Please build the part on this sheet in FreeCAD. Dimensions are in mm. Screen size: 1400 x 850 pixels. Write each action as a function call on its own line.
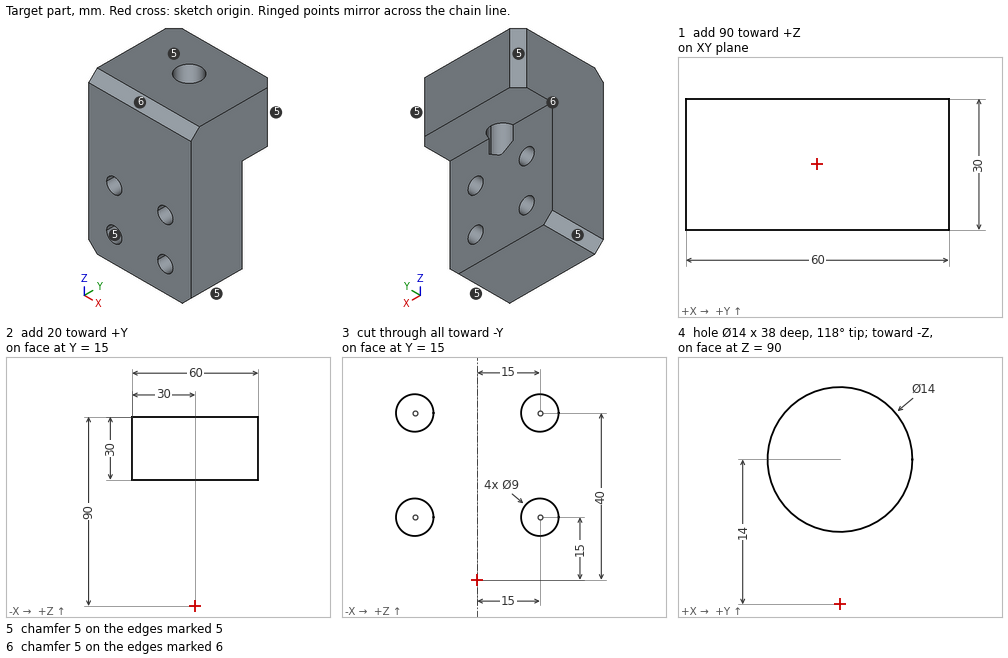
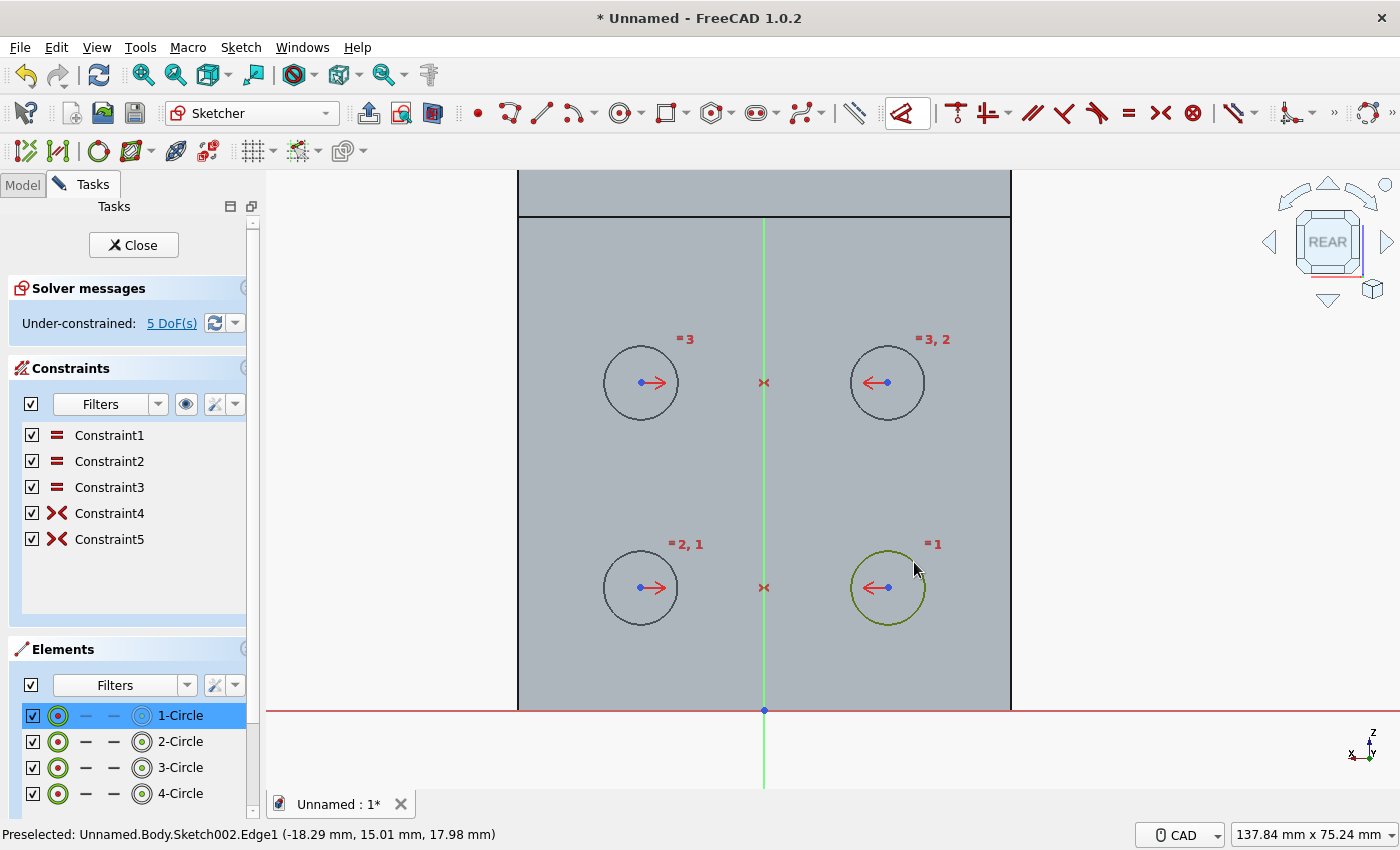
key(k)
key(o)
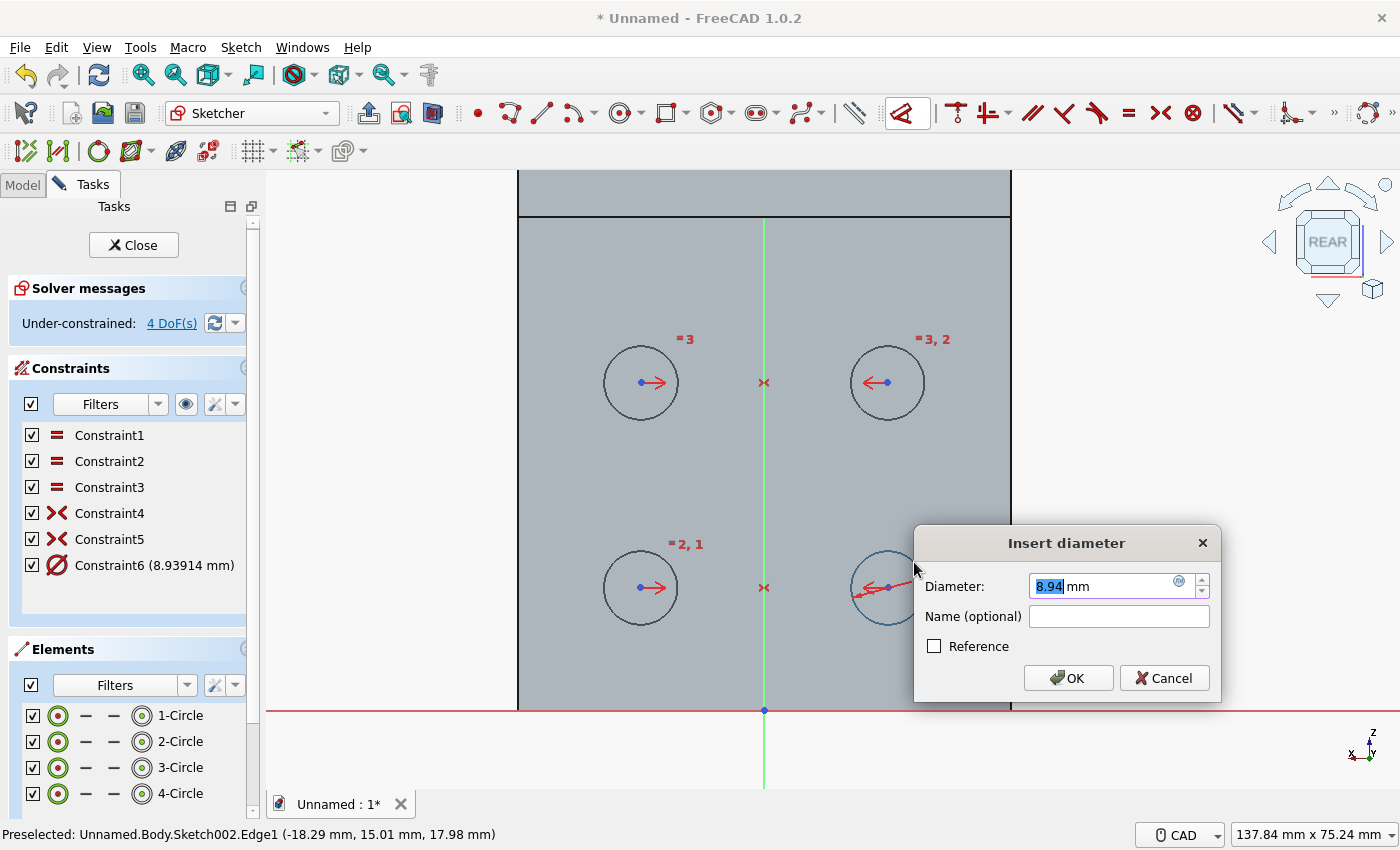
text(9)
key(Return)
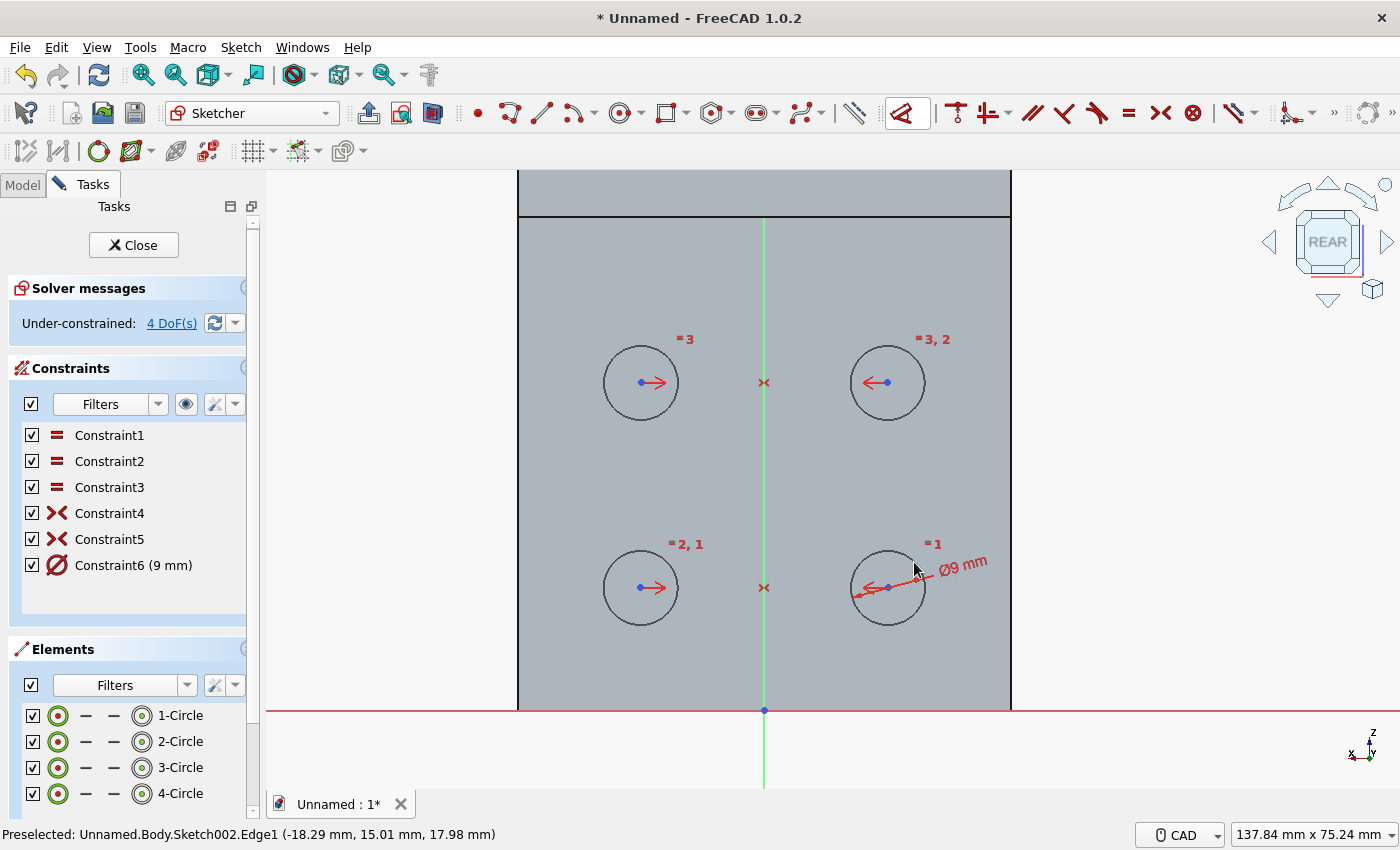
click(888, 588)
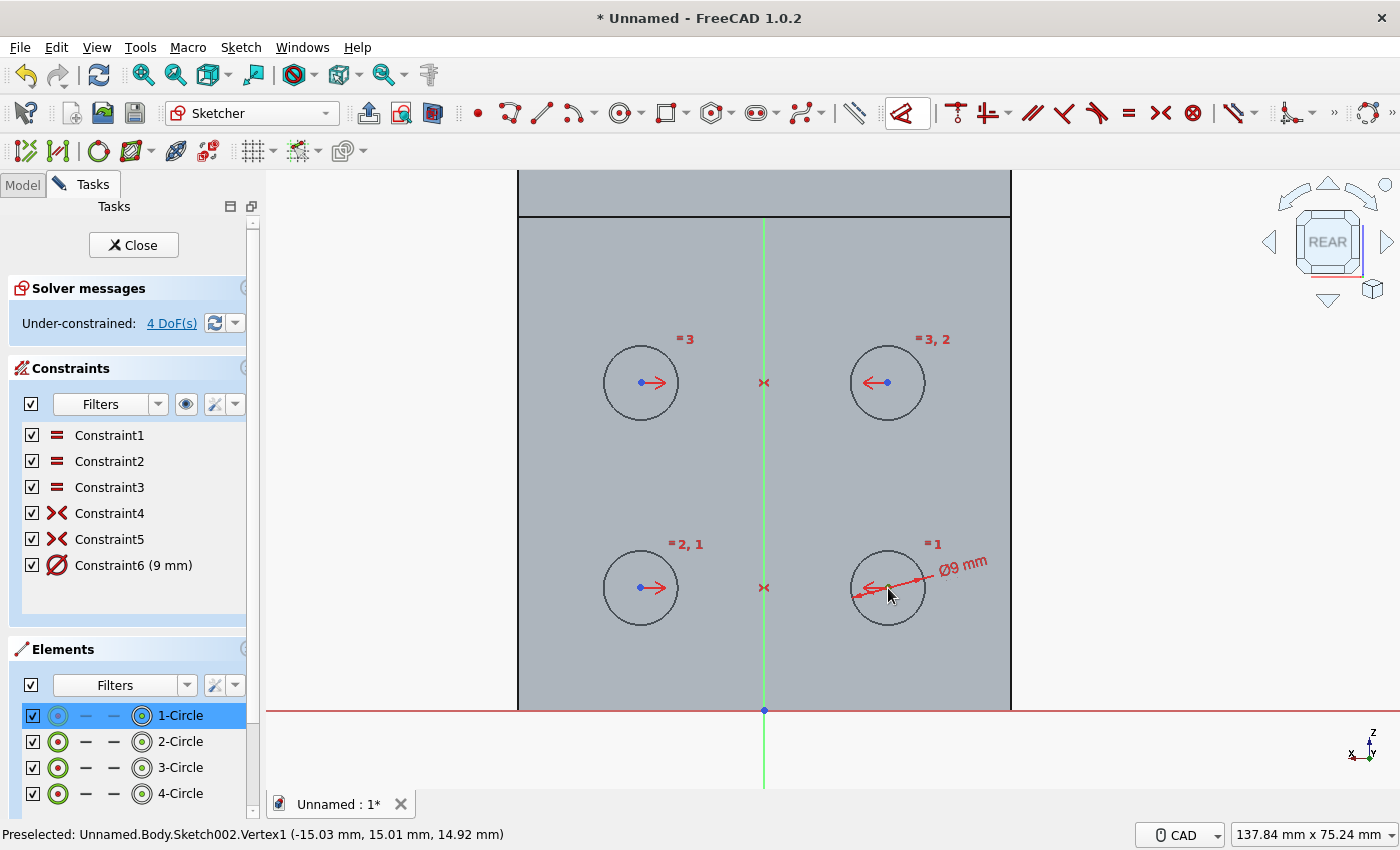
key(l)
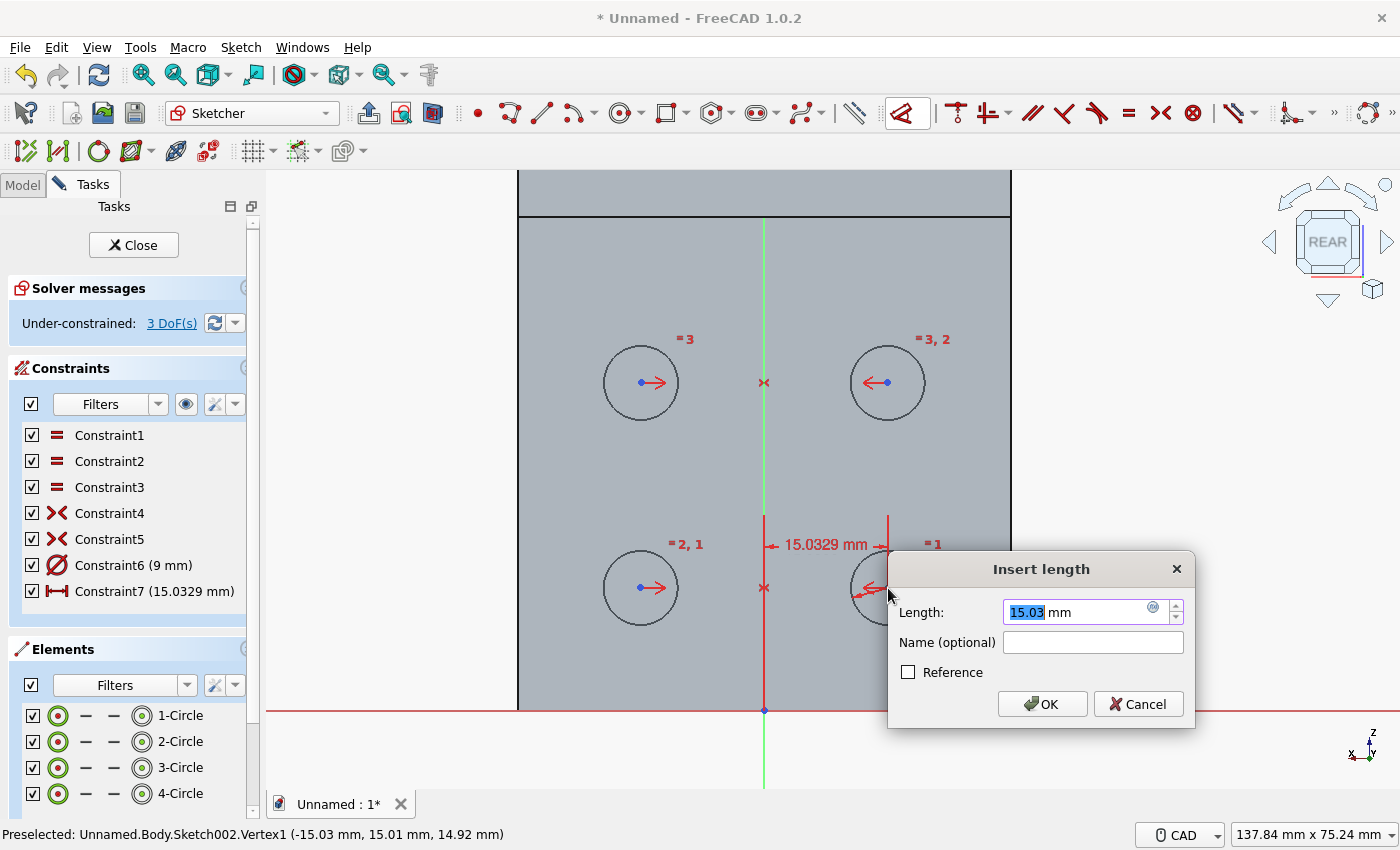
text(15)
key(Return)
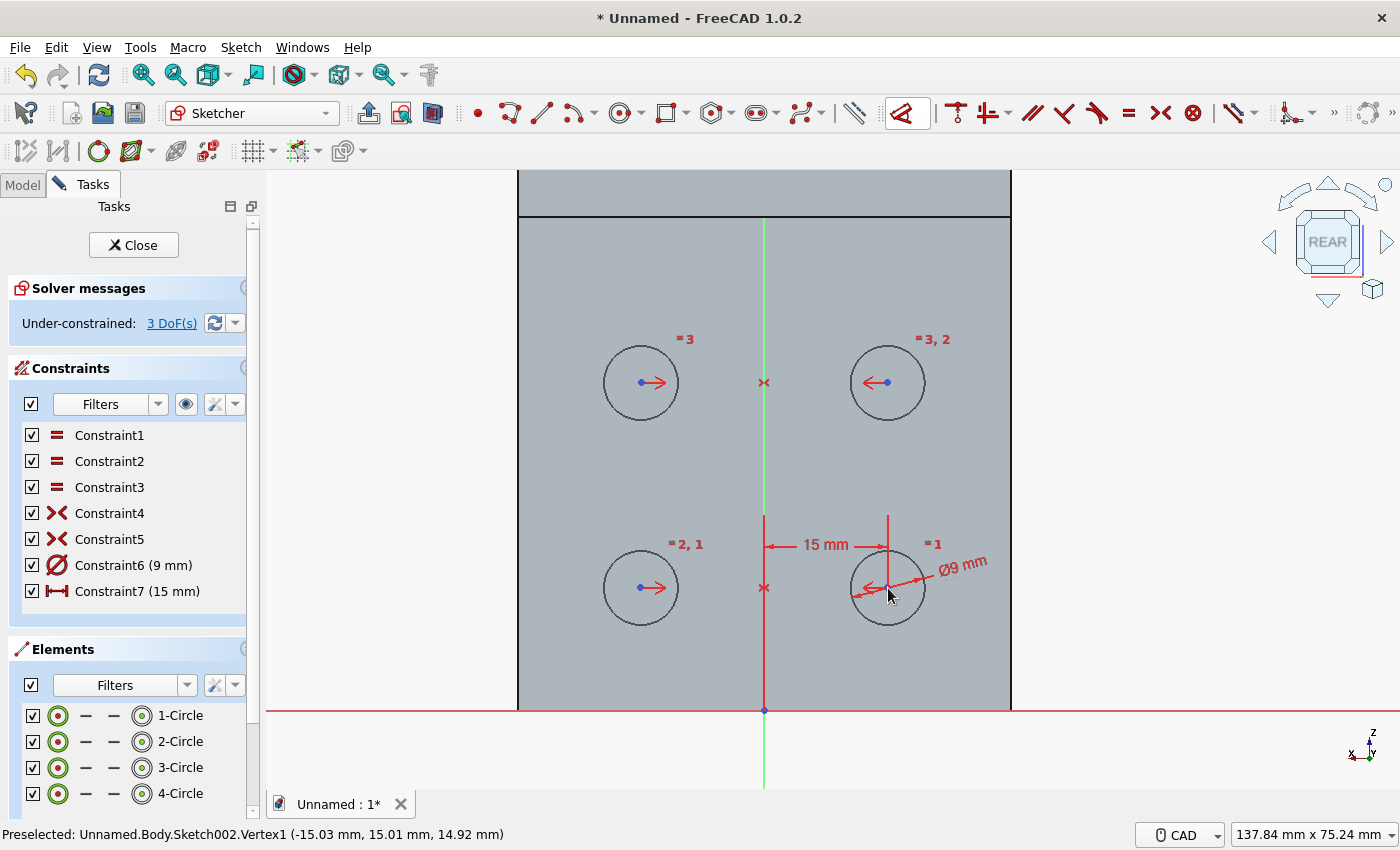
click(888, 588)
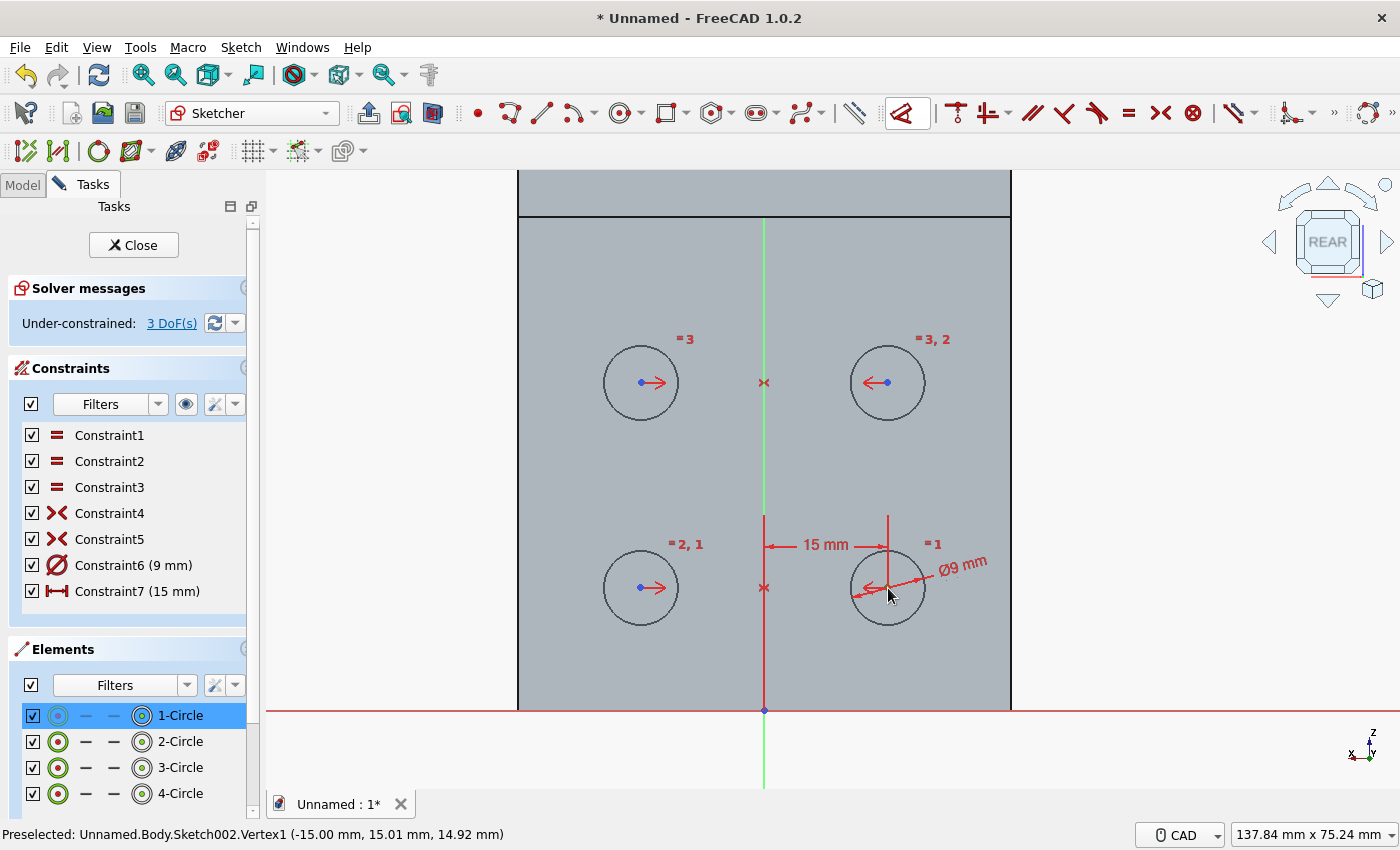
key(i)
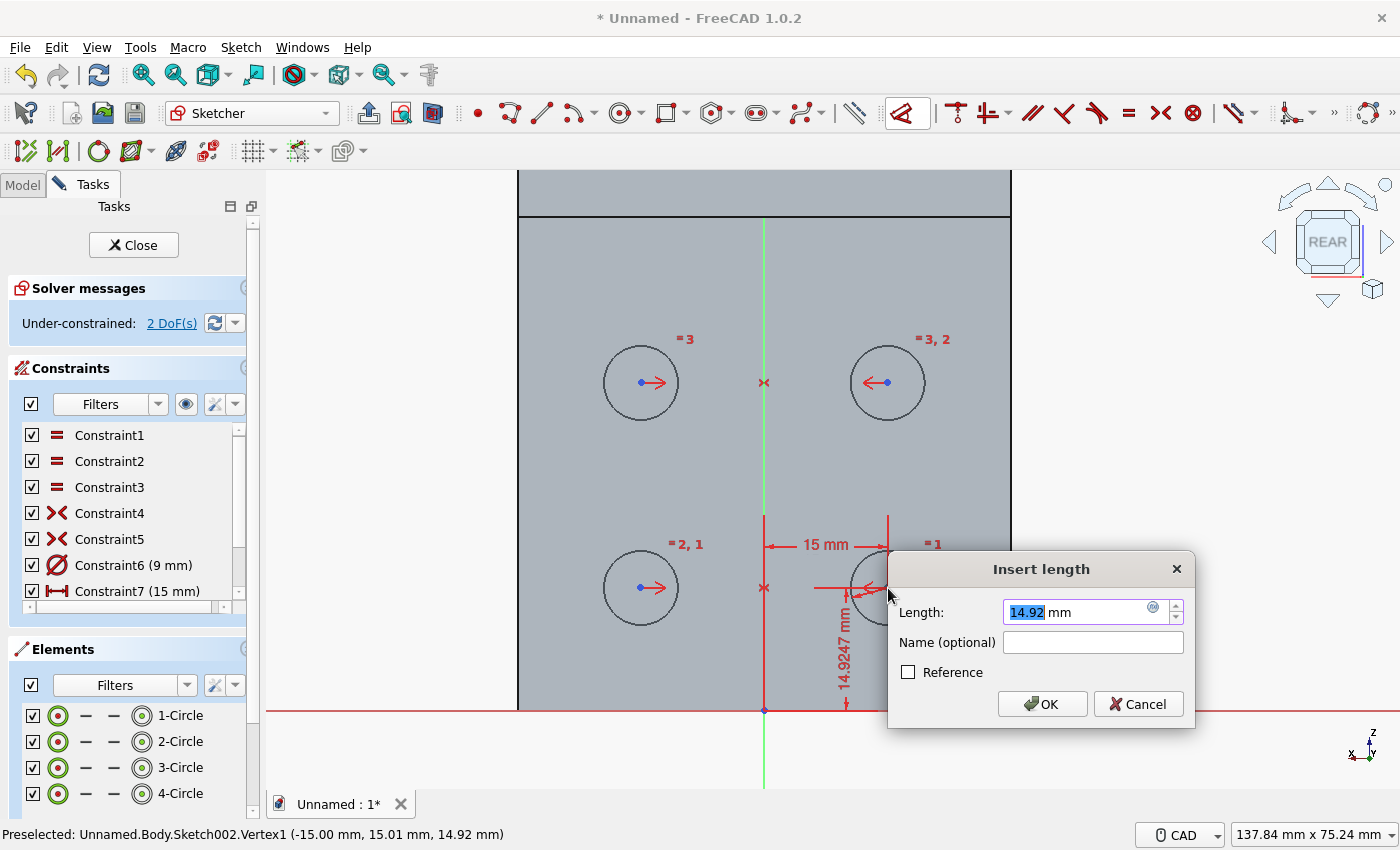
text(15)
key(Return)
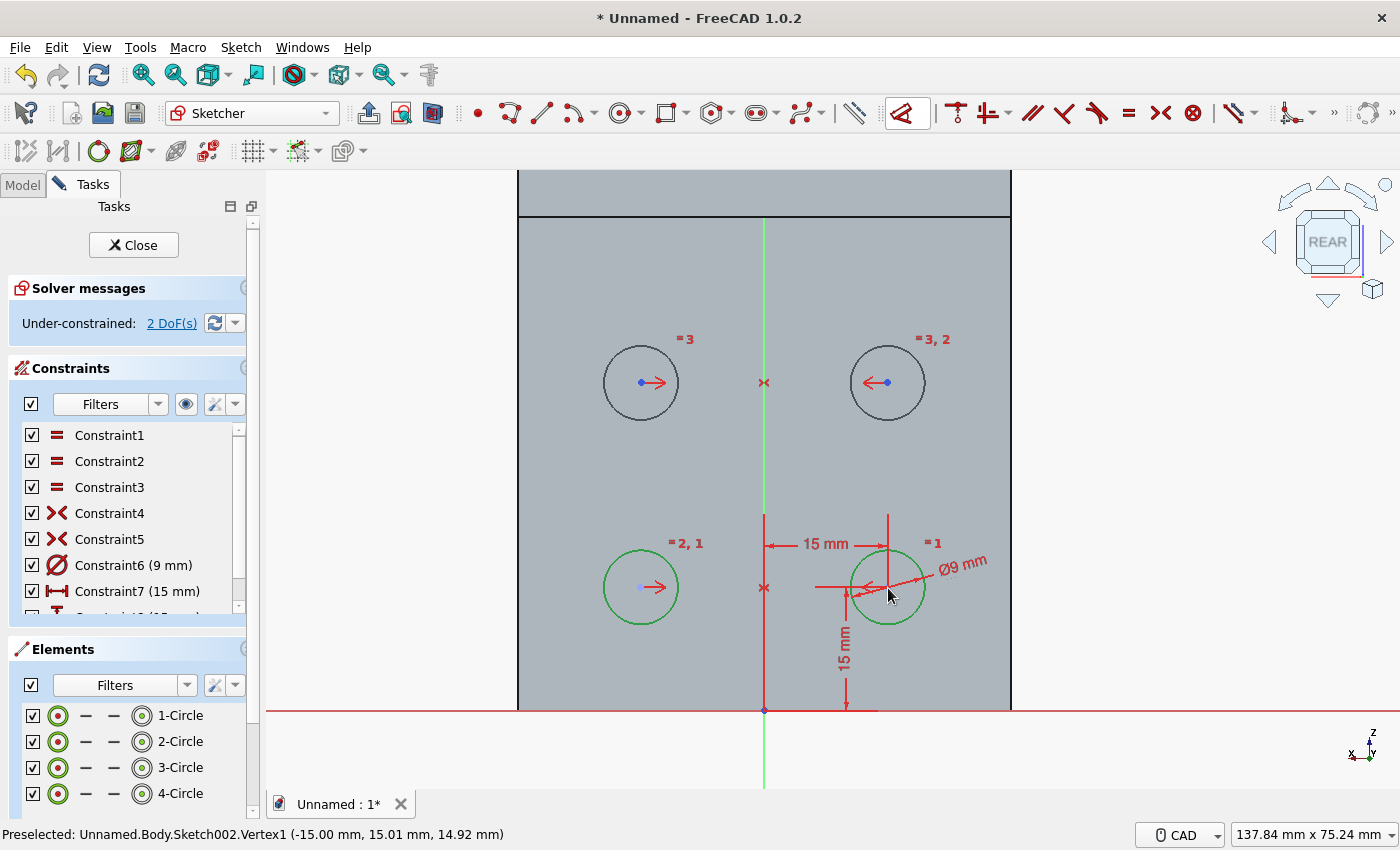
click(888, 383)